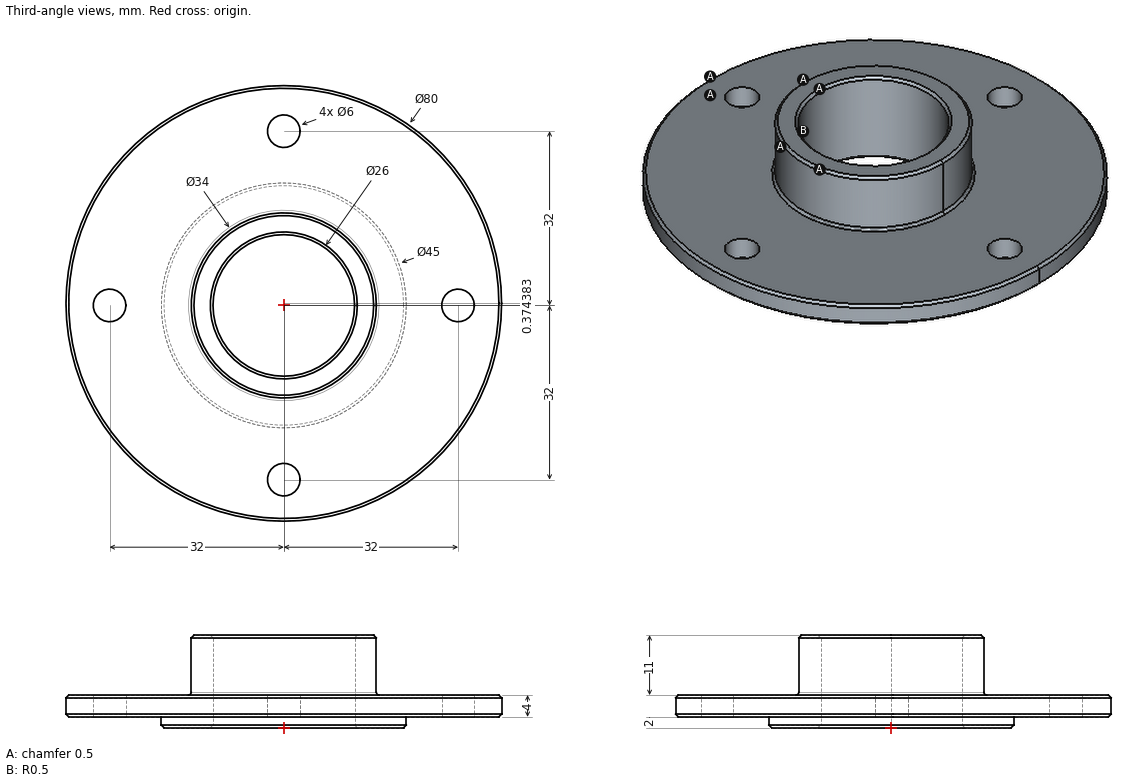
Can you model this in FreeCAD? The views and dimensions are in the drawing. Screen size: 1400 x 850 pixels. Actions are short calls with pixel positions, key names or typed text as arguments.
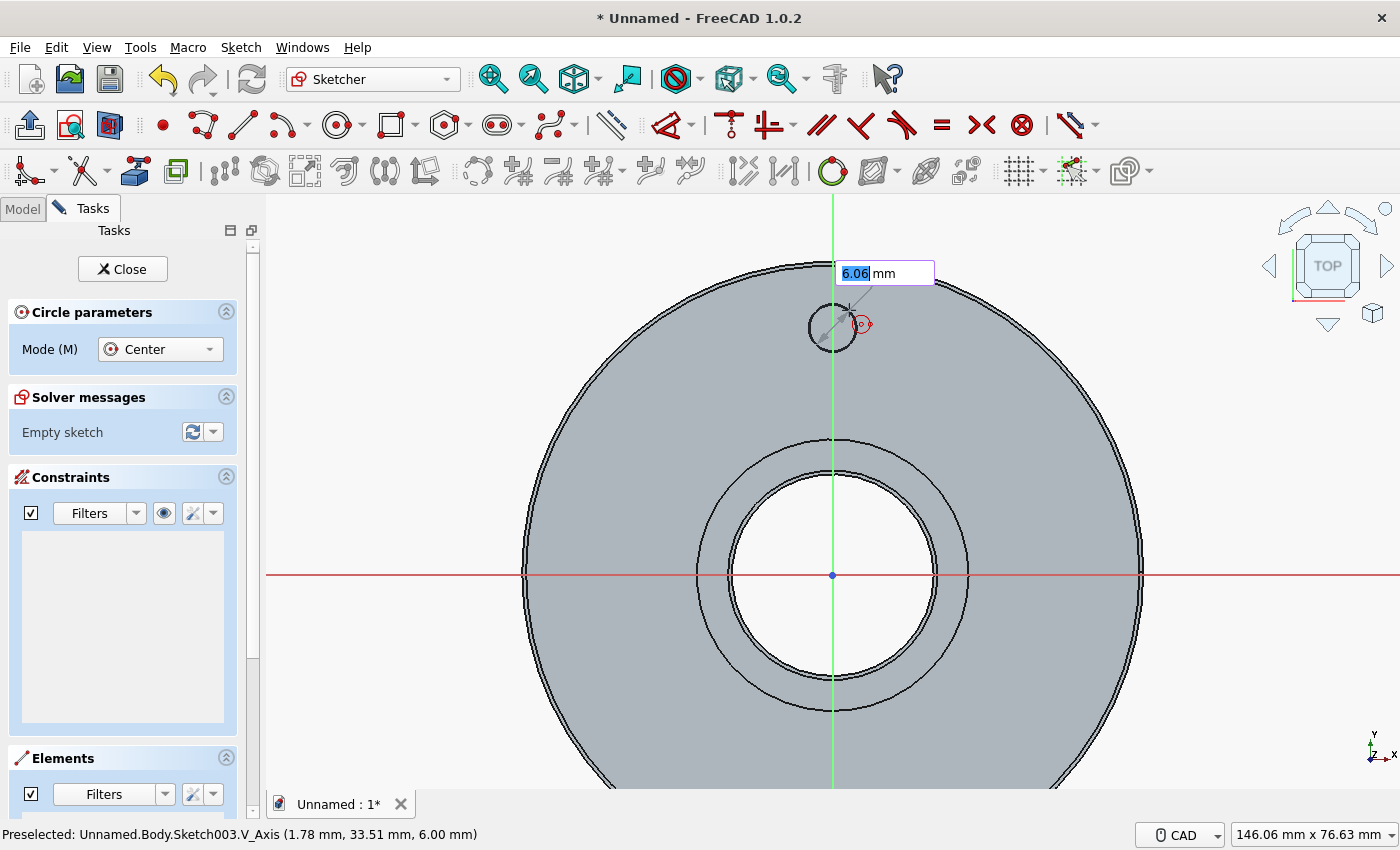
text(6)
key(Return)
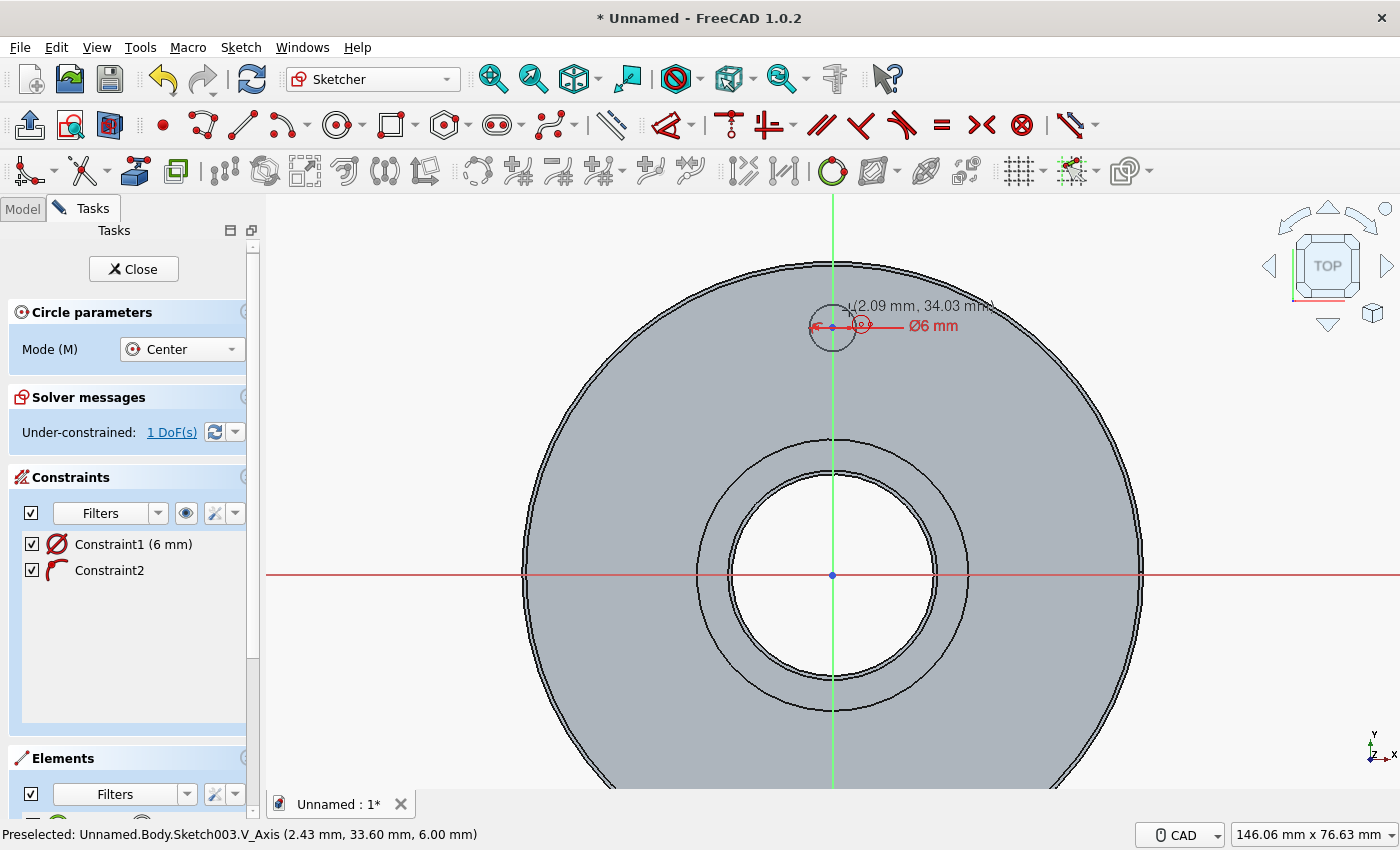
click(584, 575)
move(601, 559)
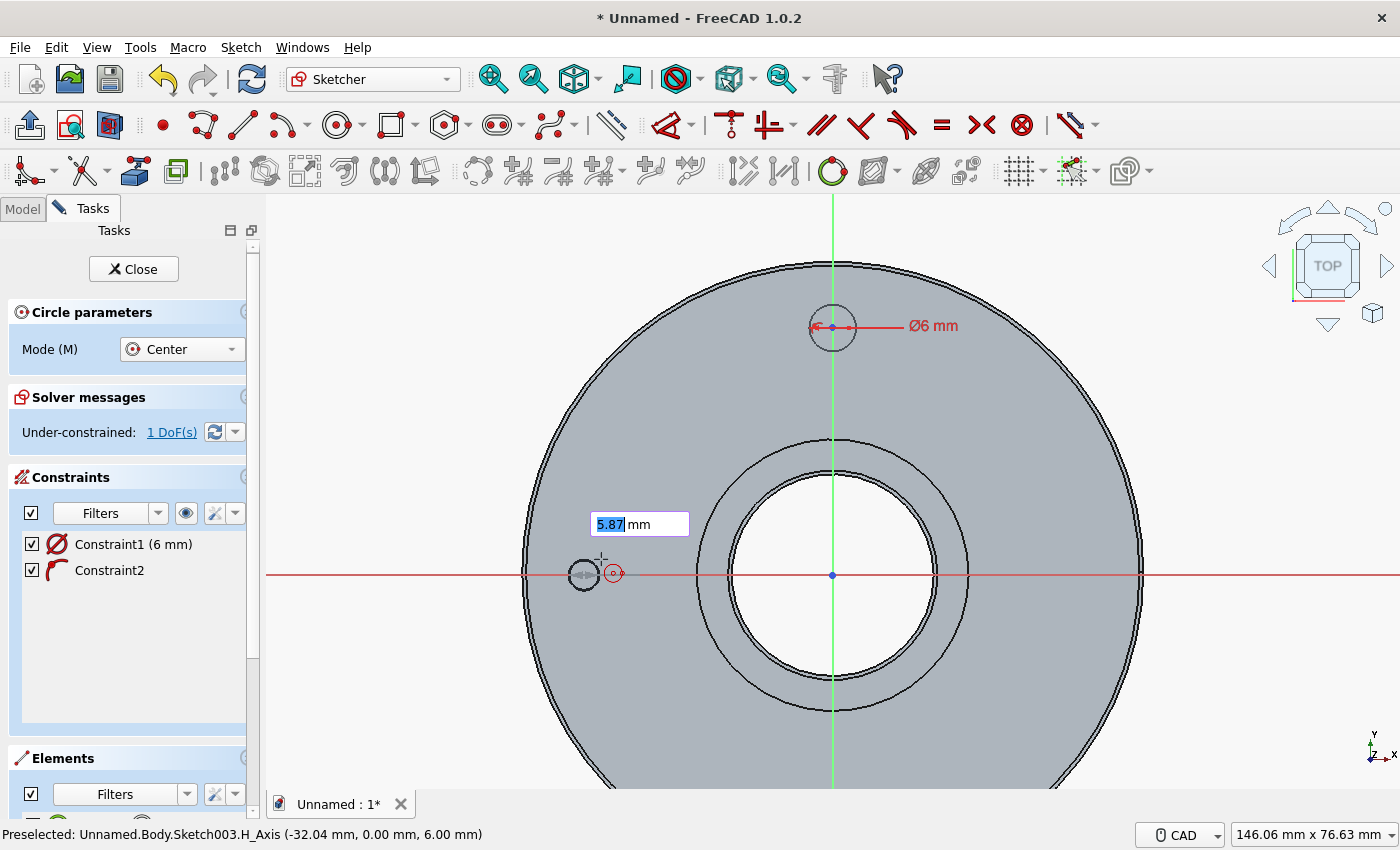
text(6)
key(Return)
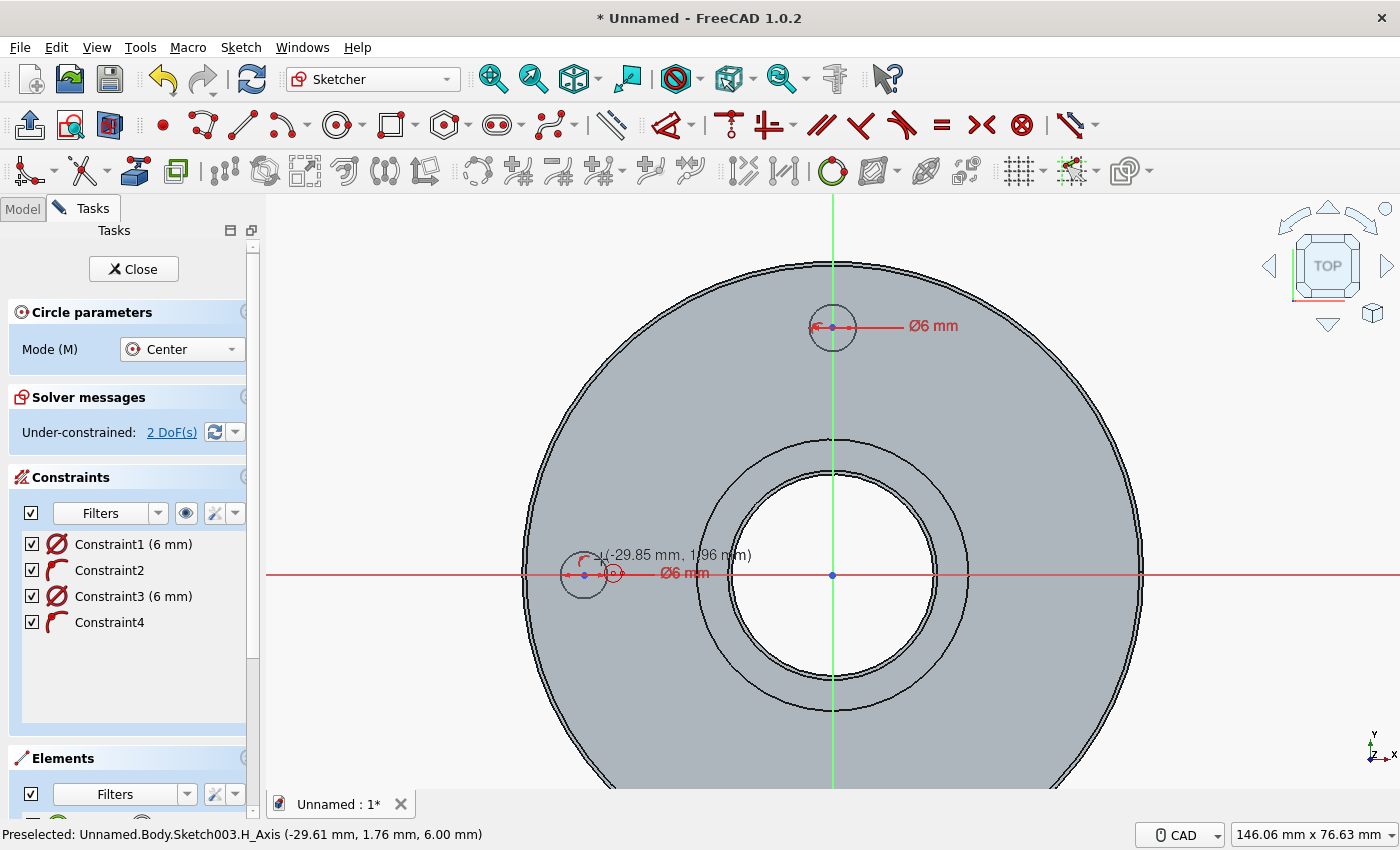
scroll(626, 321, down, 2)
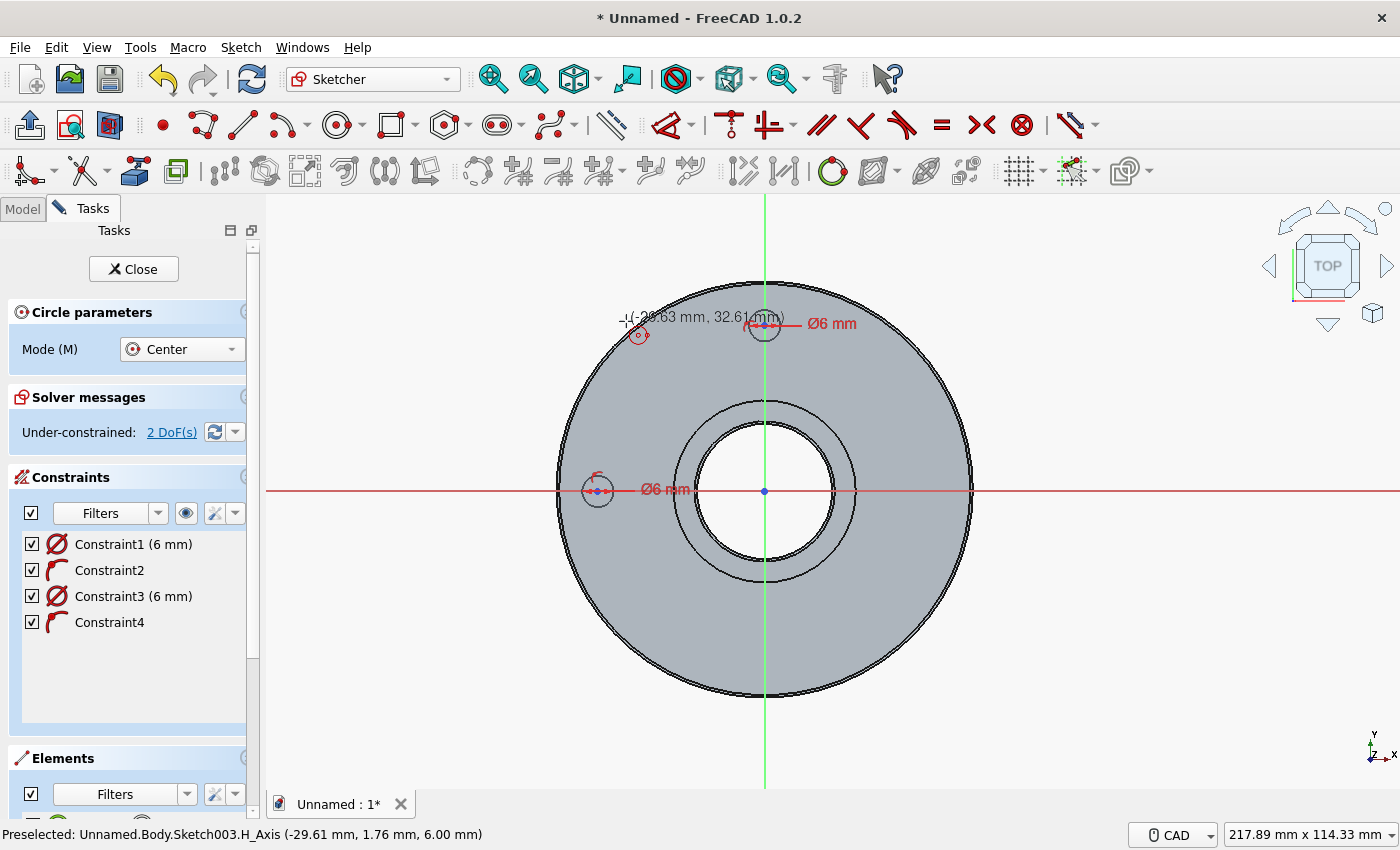
scroll(765, 658, up, 2)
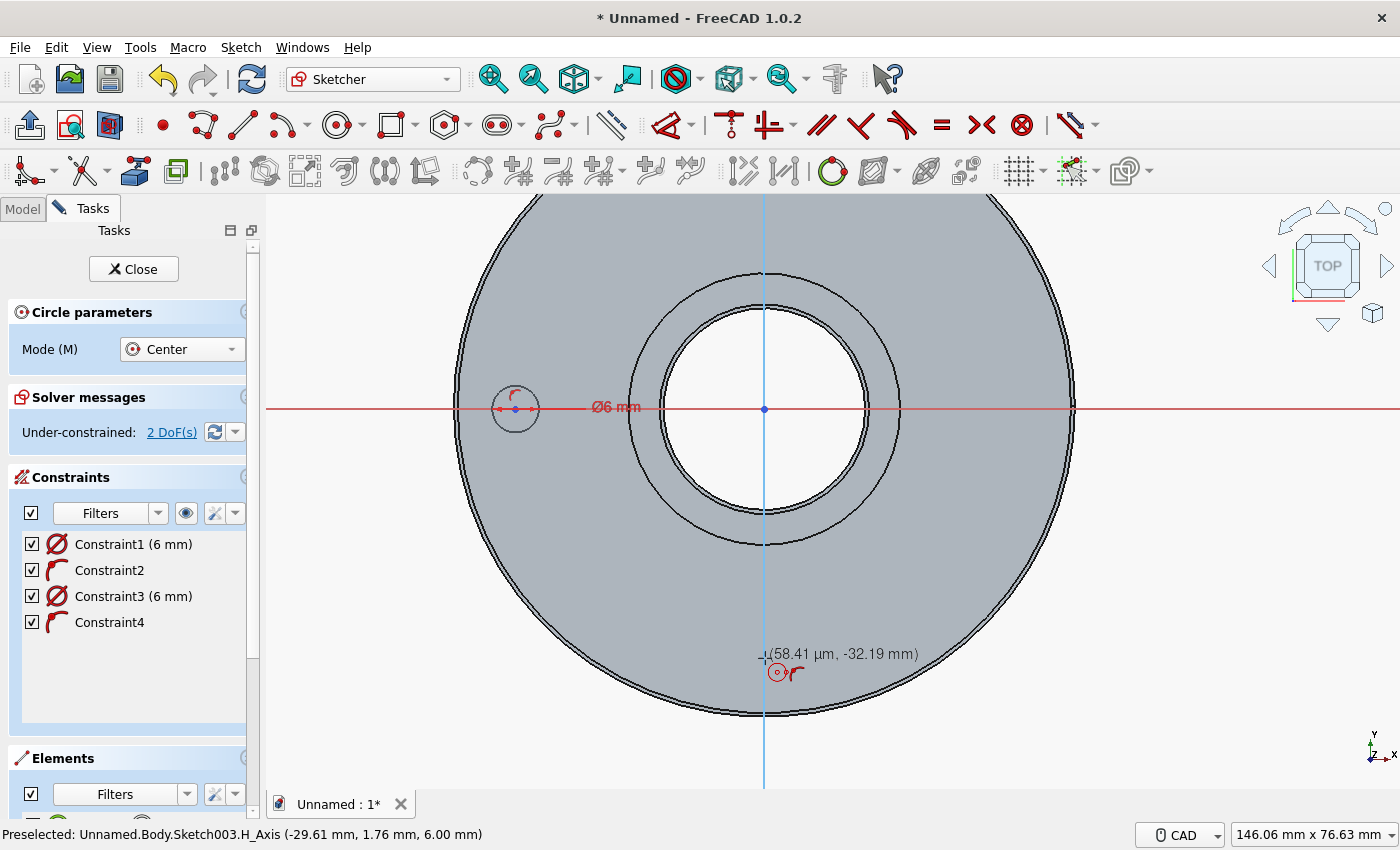
click(764, 658)
move(781, 641)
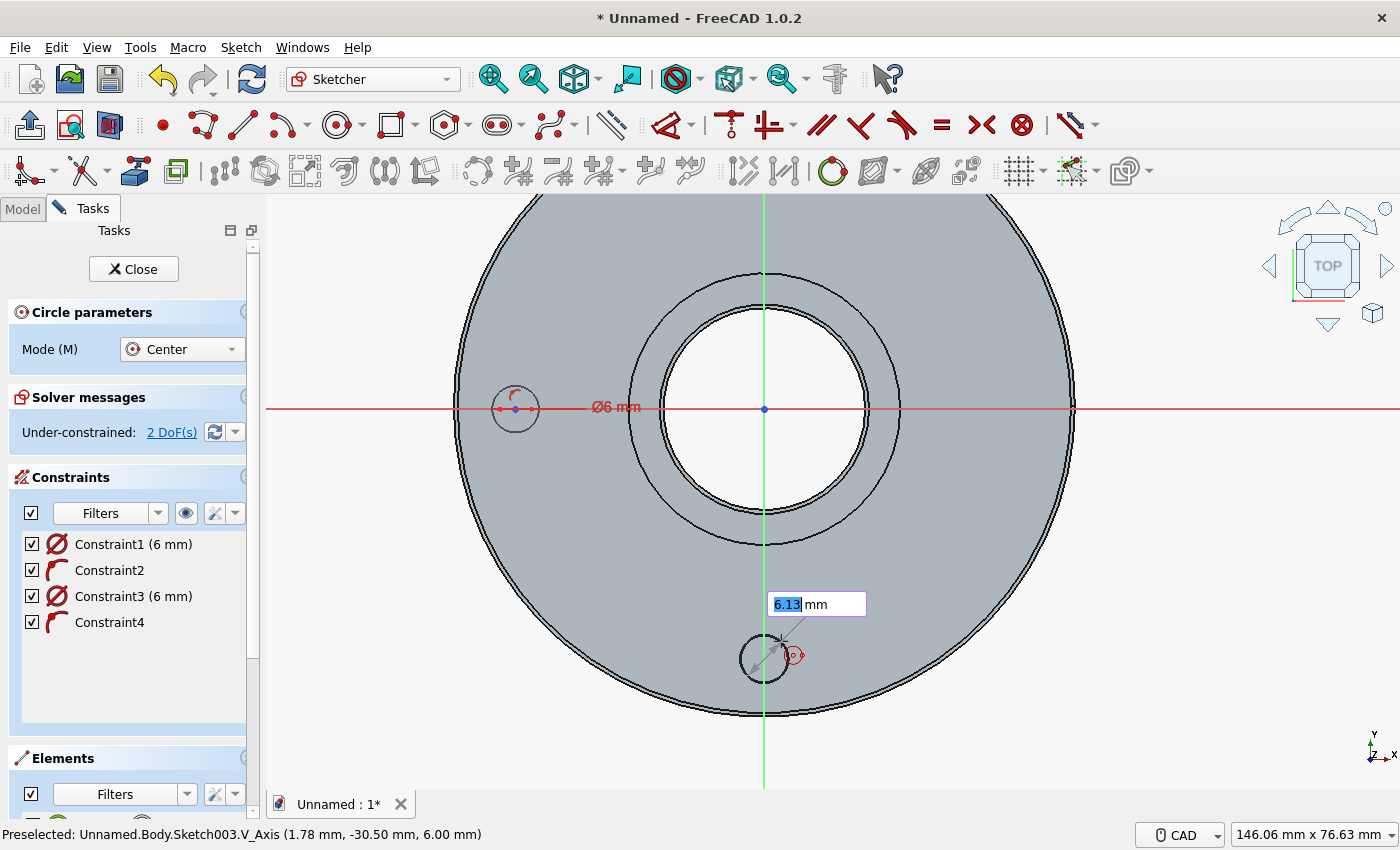
text(6)
key(Return)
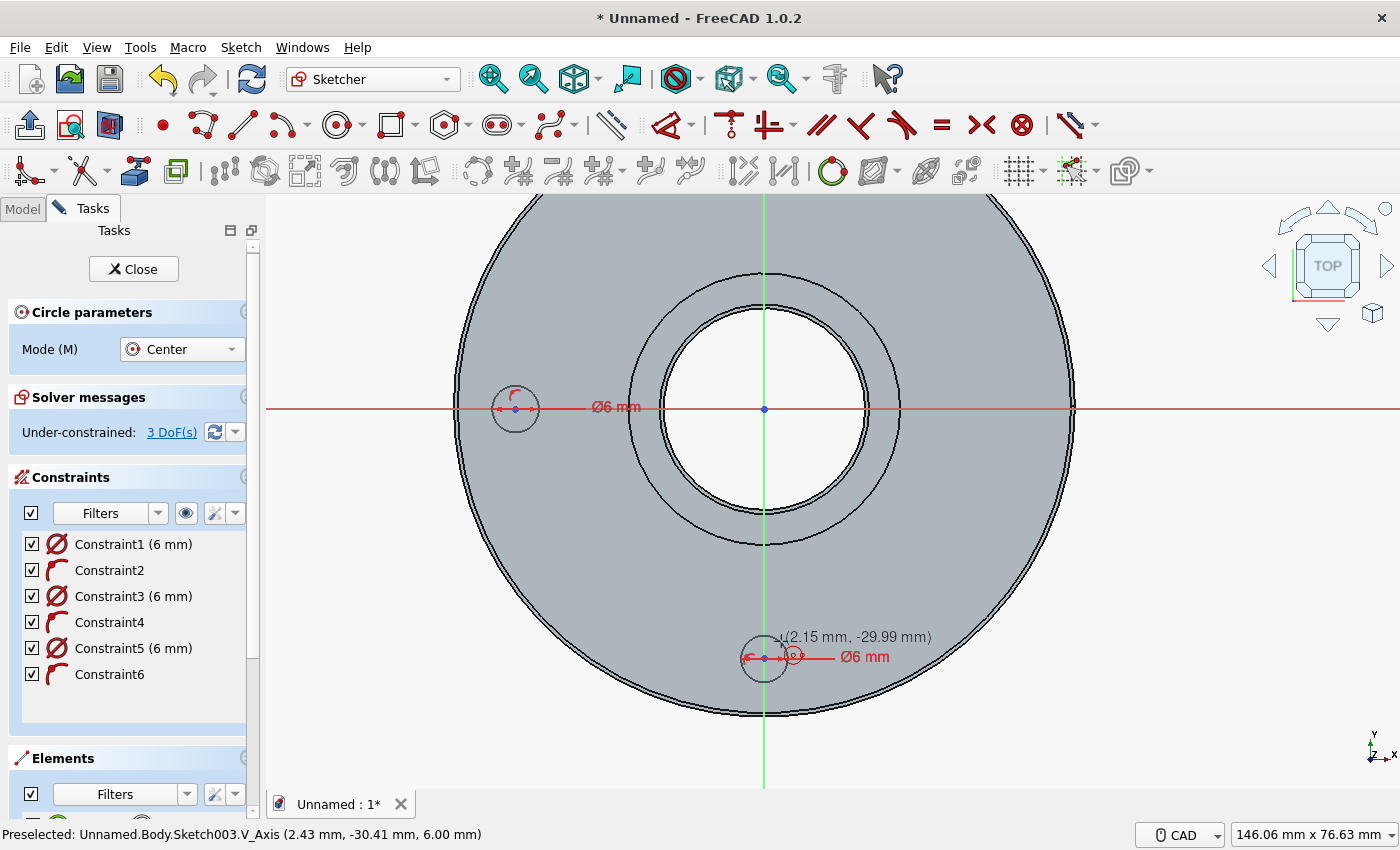
click(1013, 409)
move(1029, 393)